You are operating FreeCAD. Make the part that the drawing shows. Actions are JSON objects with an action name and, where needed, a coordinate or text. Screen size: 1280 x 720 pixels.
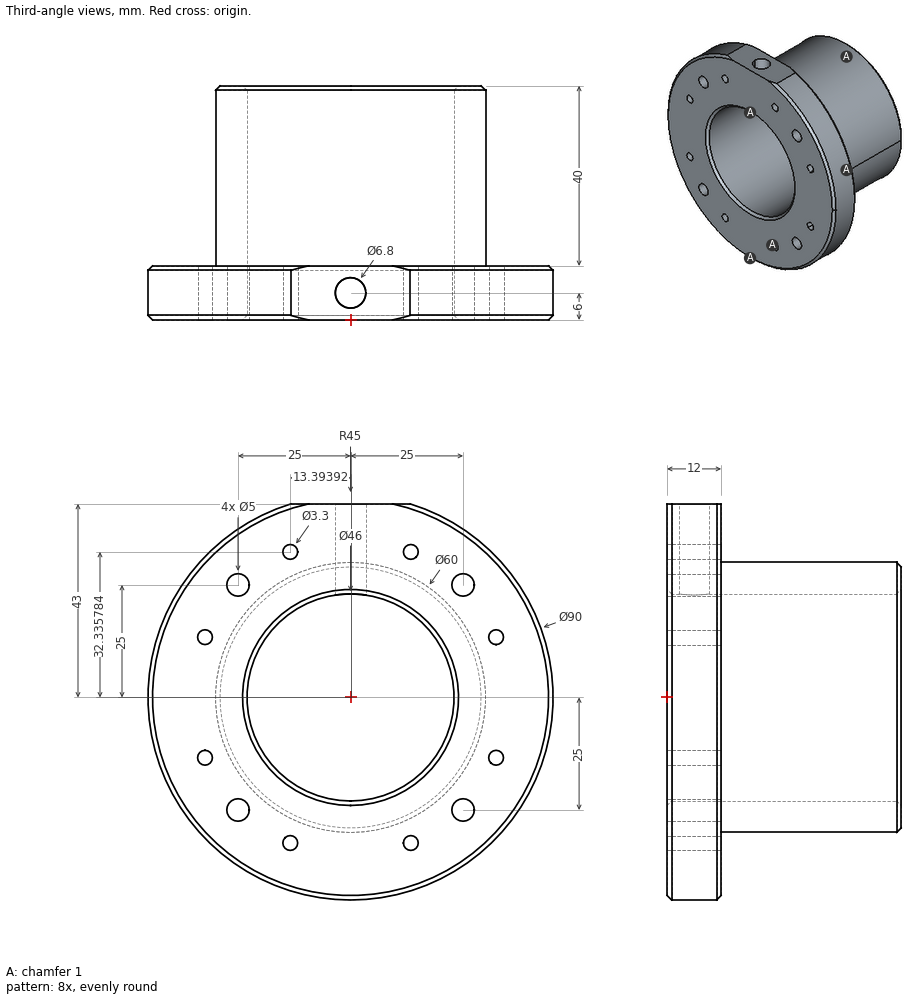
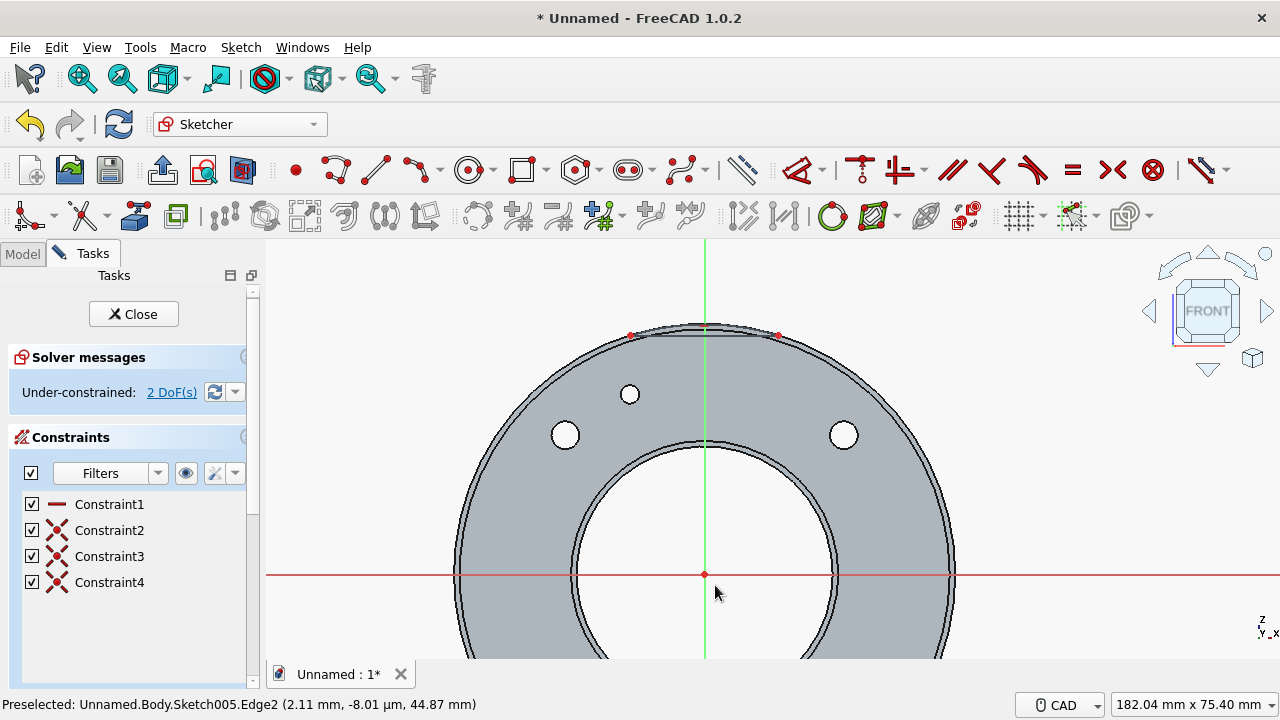
{"action": "key", "text": "d"}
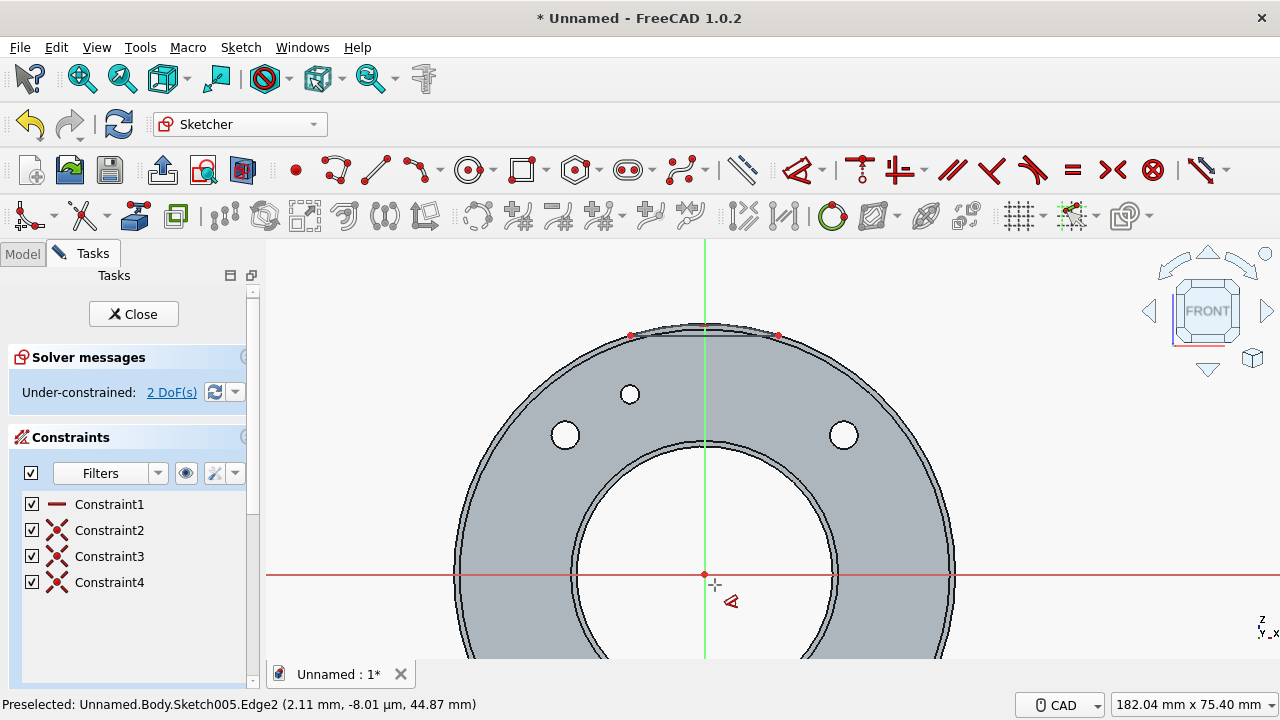
{"action": "scroll", "coordinate": [735, 326], "scroll_direction": "up", "scroll_amount": 2}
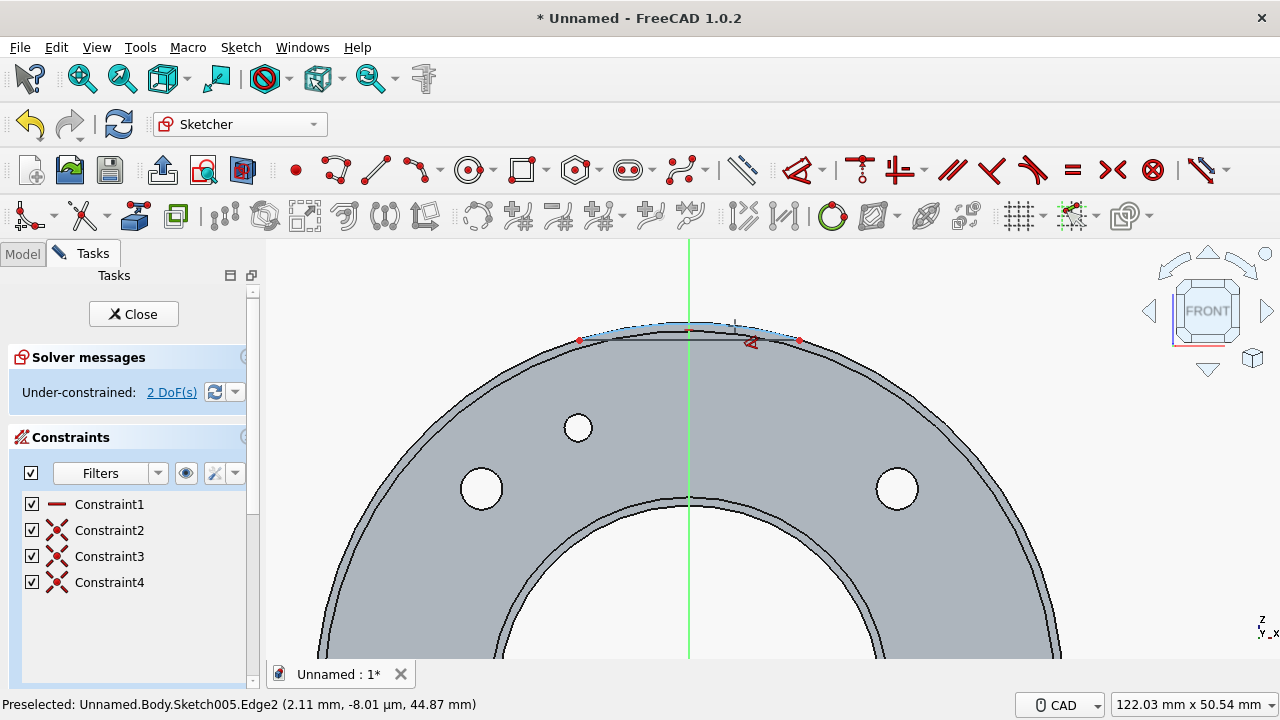
{"action": "left_click", "coordinate": [734, 326]}
{"action": "left_click", "coordinate": [738, 294]}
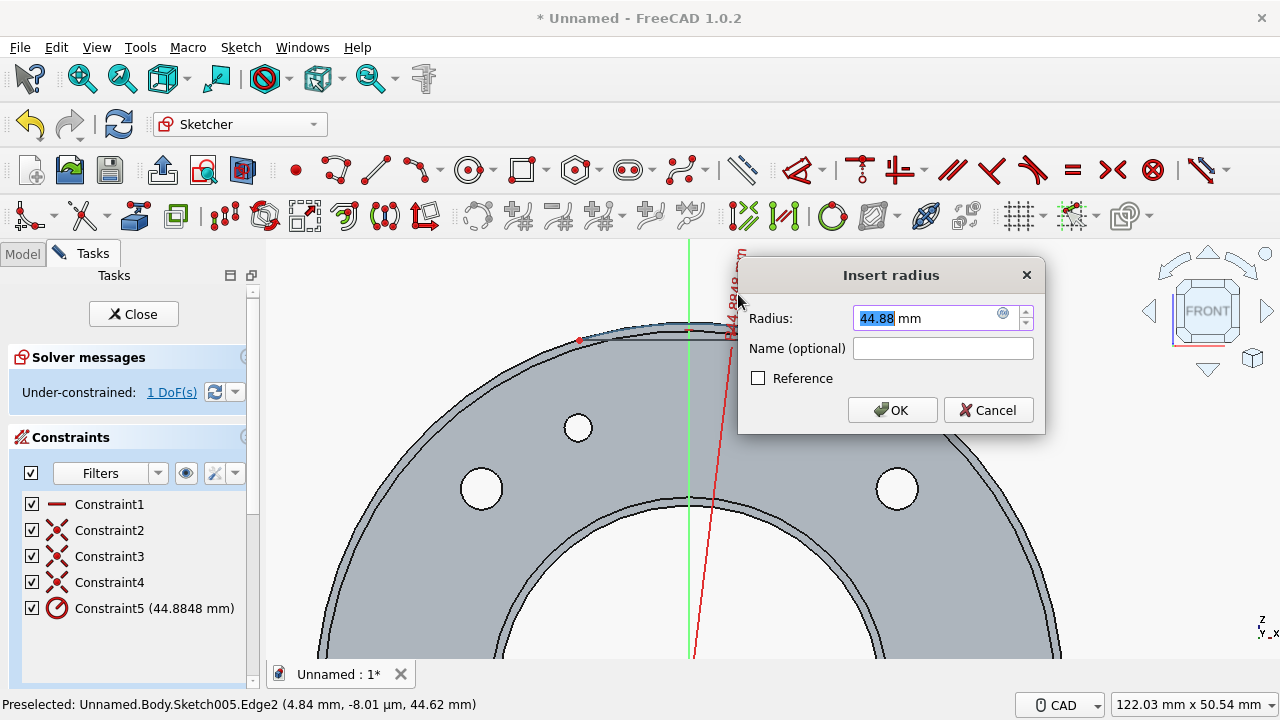
{"action": "type", "text": "45"}
{"action": "key", "text": "Return"}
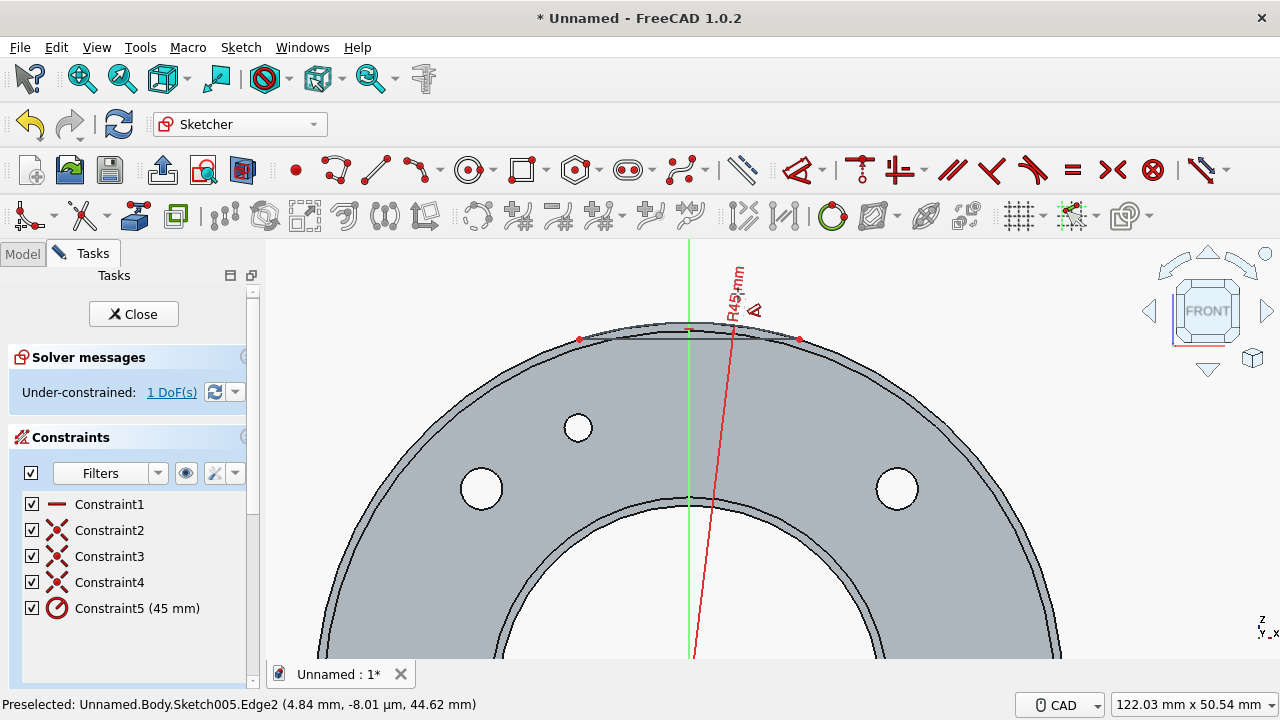
{"action": "left_click", "coordinate": [579, 339]}
{"action": "left_click", "coordinate": [545, 485]}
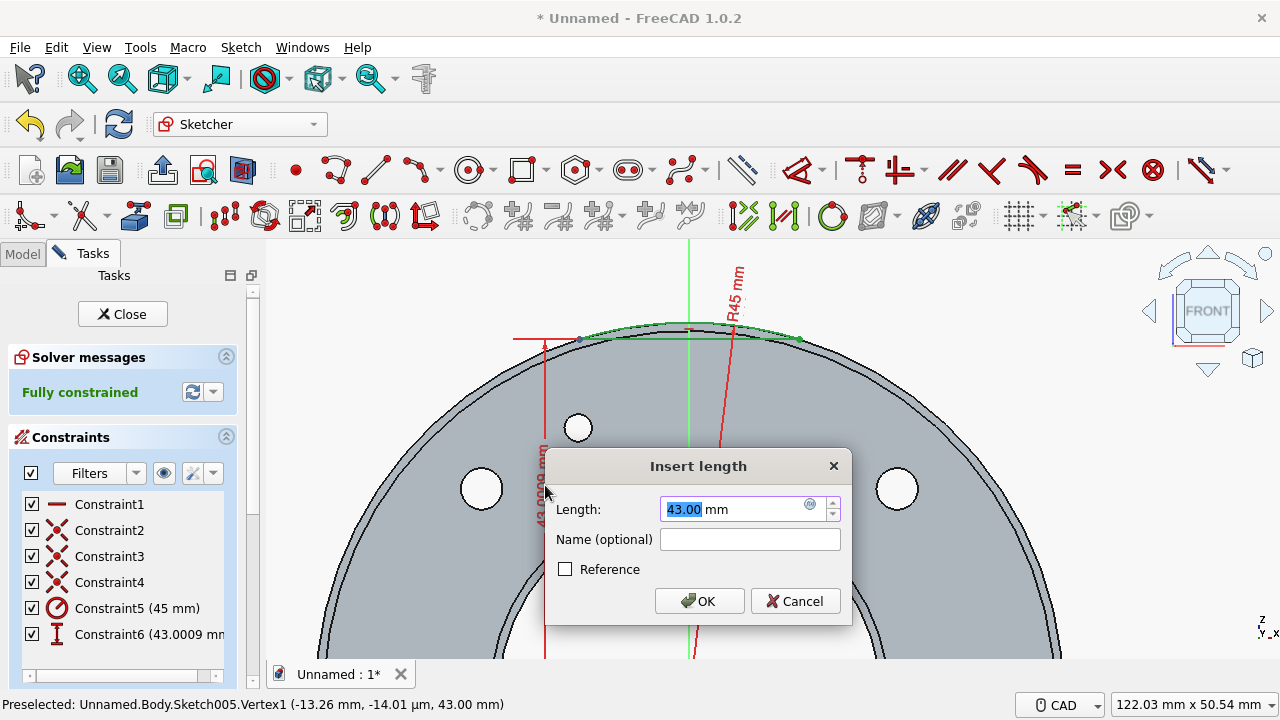
{"action": "type", "text": "43"}
{"action": "key", "text": "Return"}
{"action": "key", "text": "Escape"}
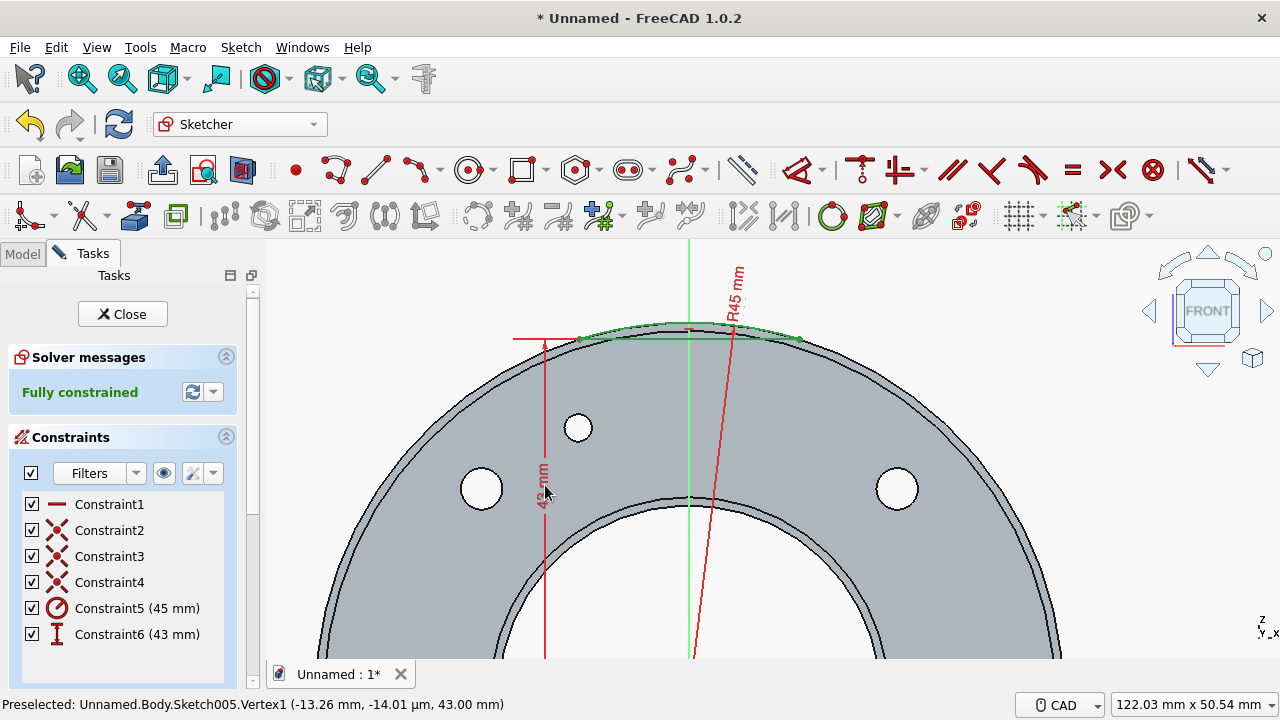
{"action": "left_click", "coordinate": [123, 314]}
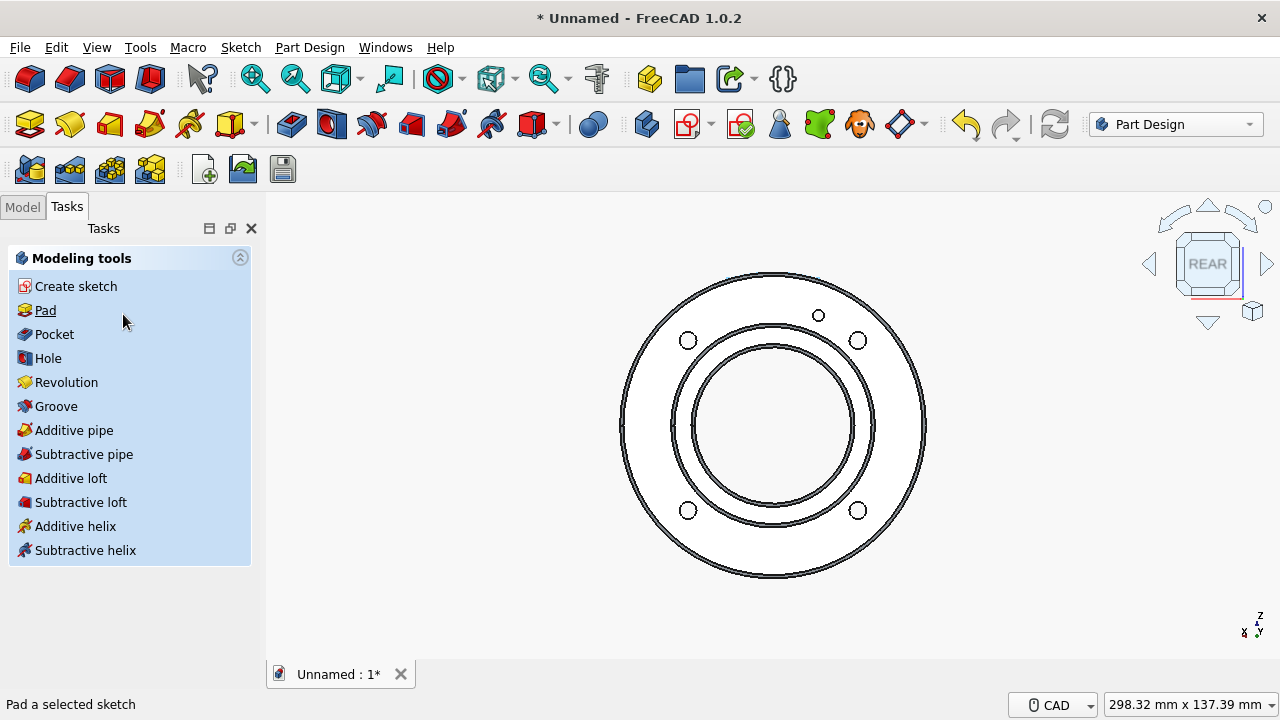
{"action": "left_click", "coordinate": [292, 124]}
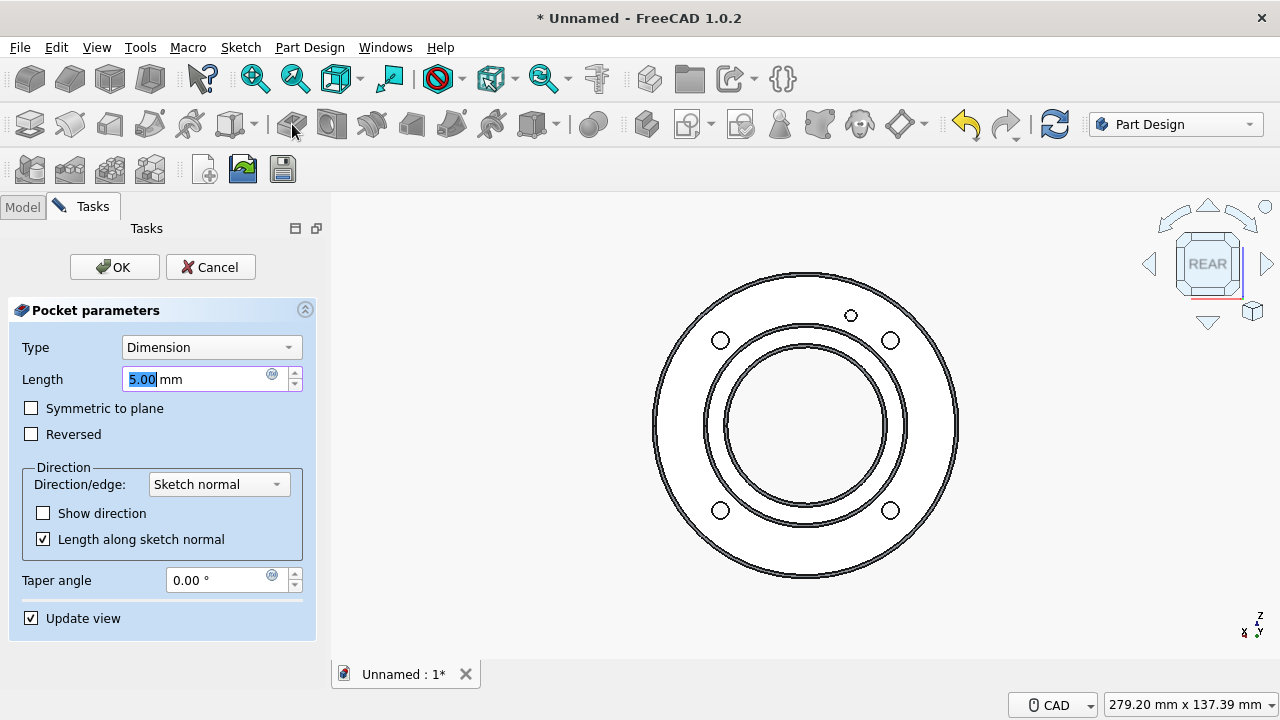
{"action": "left_click", "coordinate": [212, 348]}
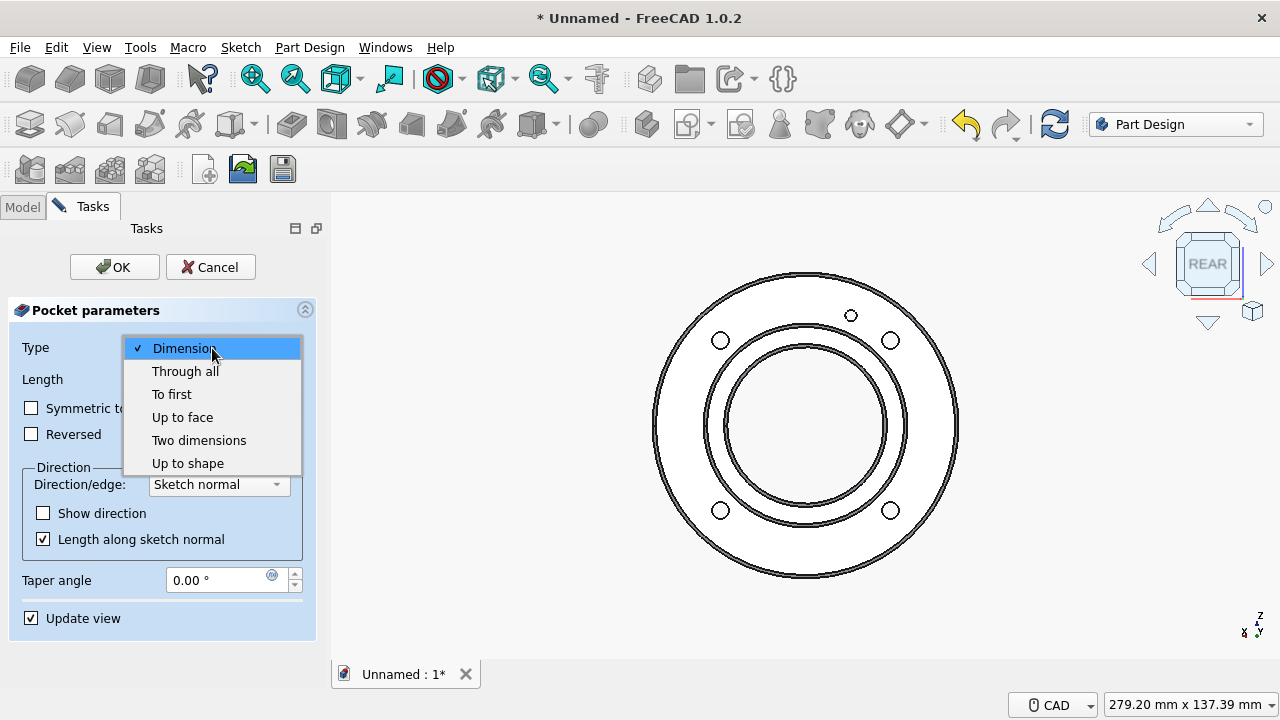
{"action": "left_click", "coordinate": [212, 372]}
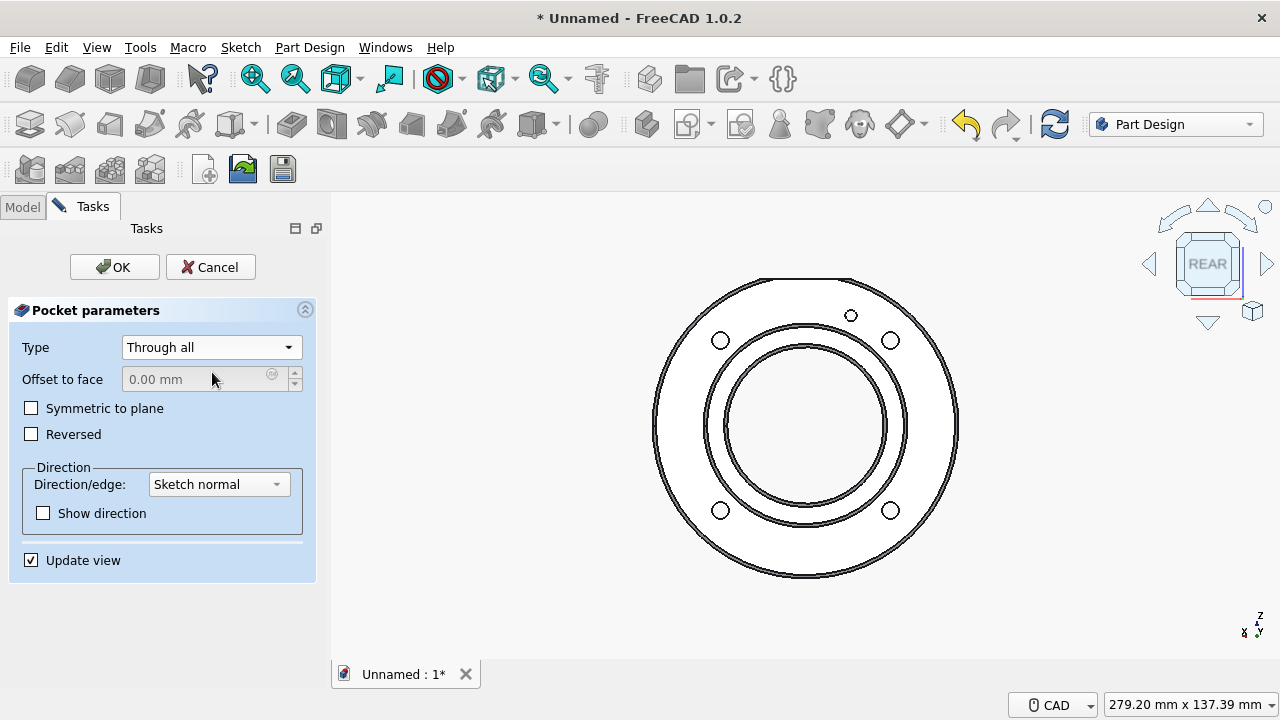
{"action": "left_click", "coordinate": [115, 267]}